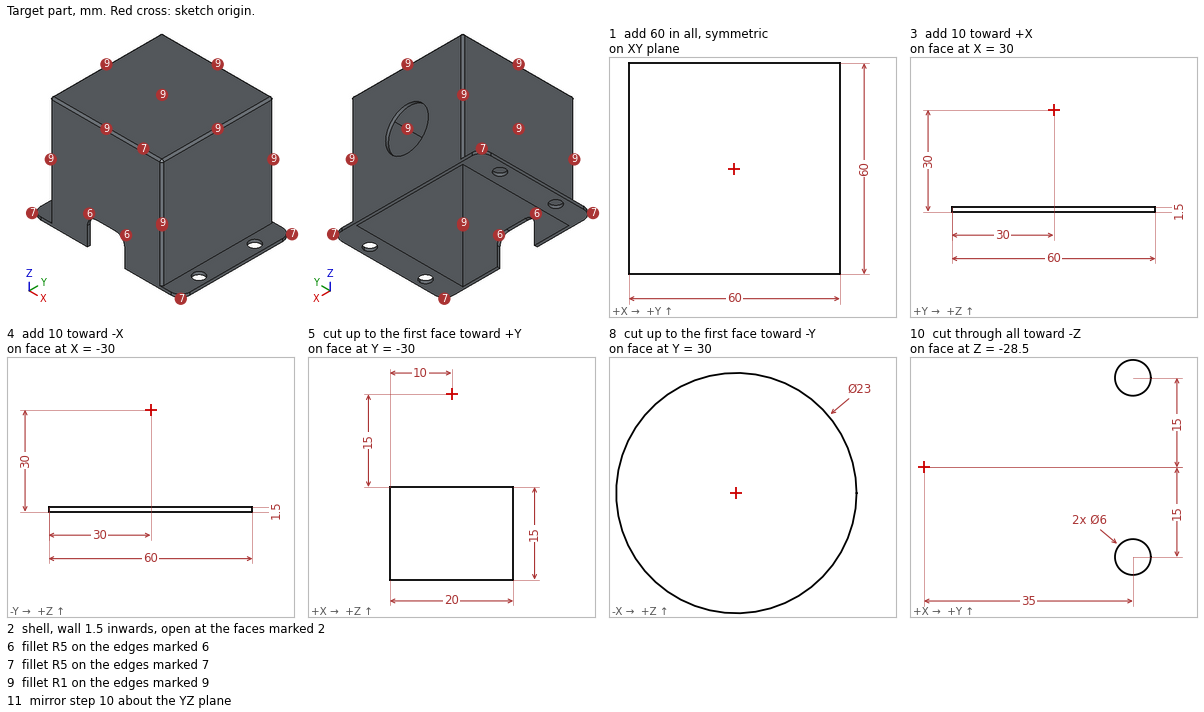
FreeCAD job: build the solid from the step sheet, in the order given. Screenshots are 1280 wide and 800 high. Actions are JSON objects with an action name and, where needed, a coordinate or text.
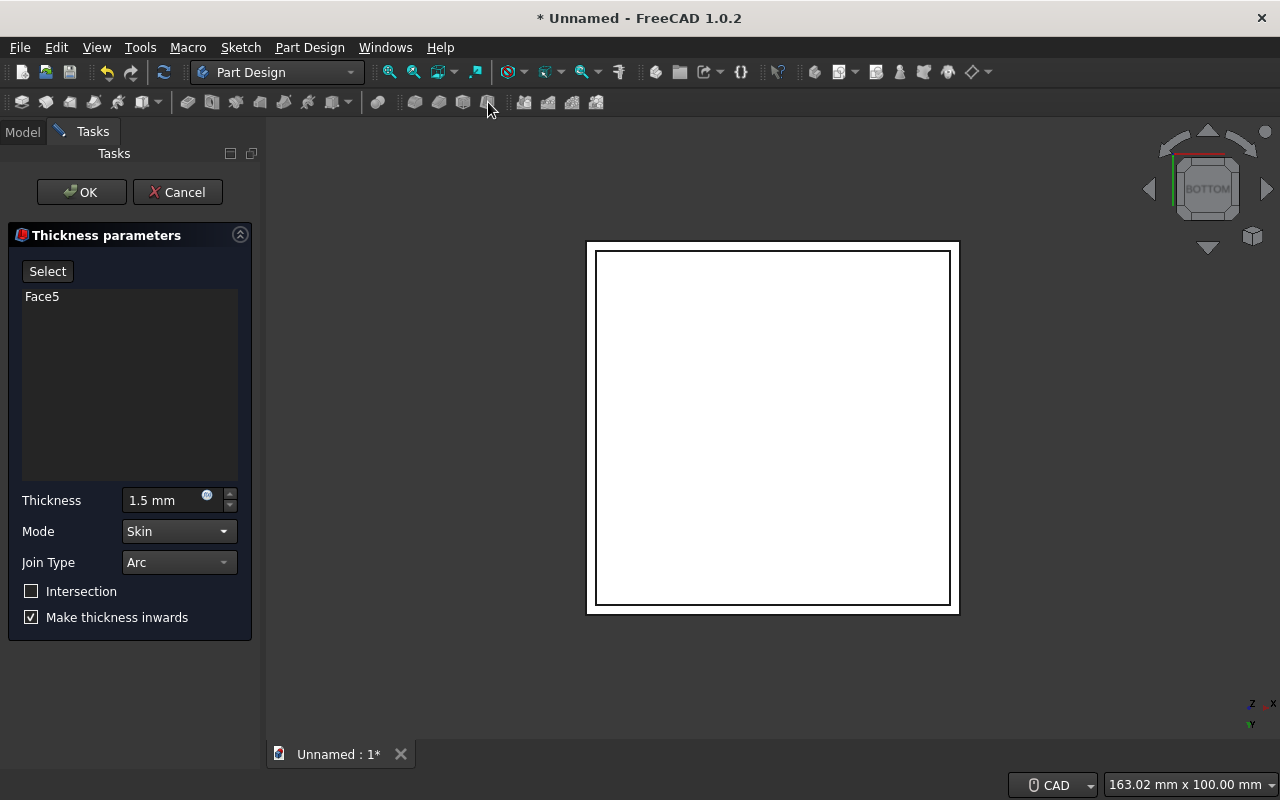
{"action": "left_click", "coordinate": [180, 562]}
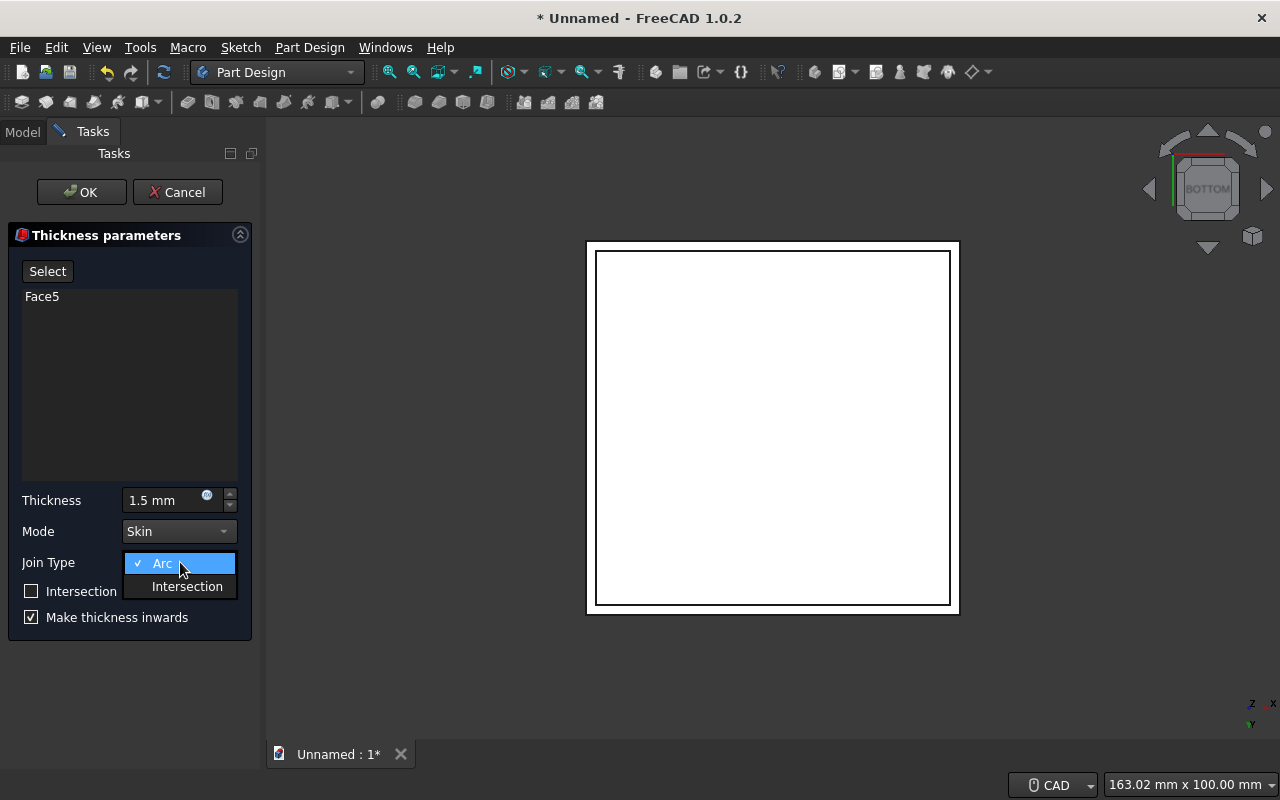
{"action": "left_click", "coordinate": [179, 586]}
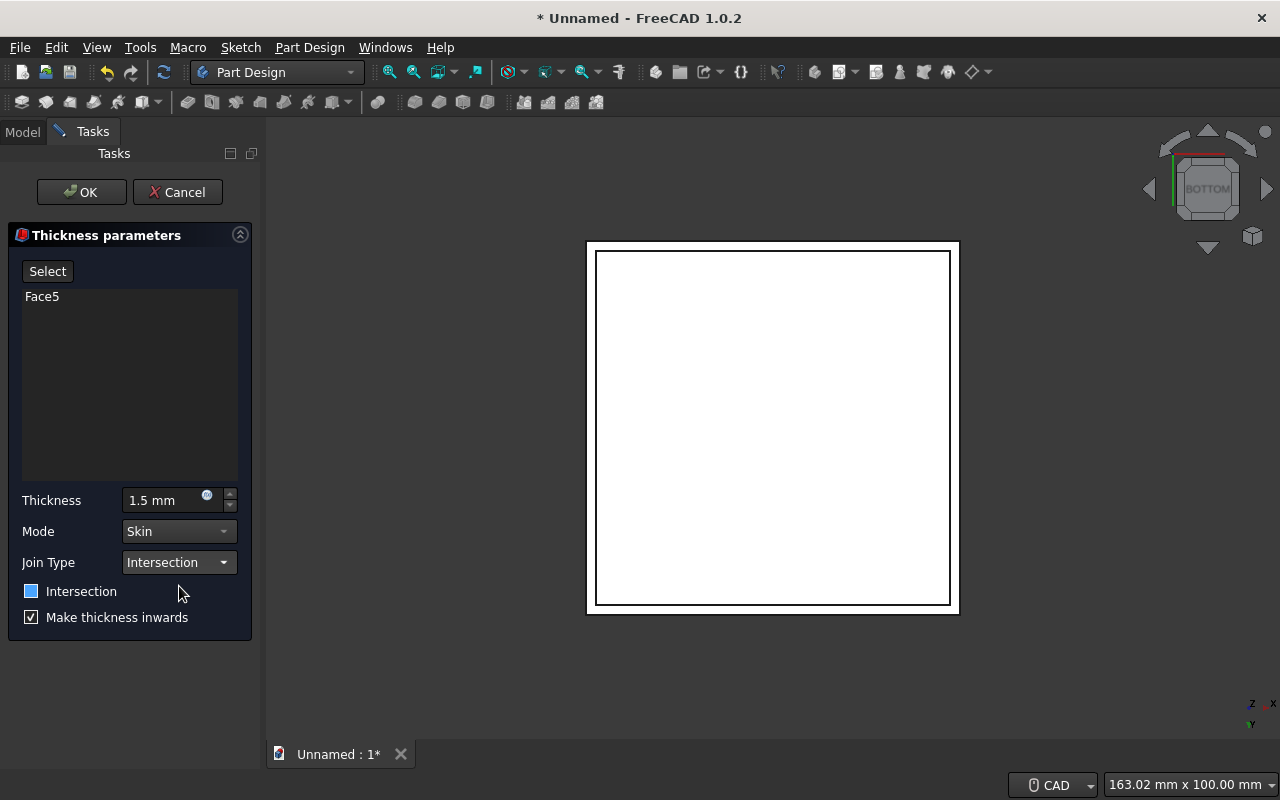
{"action": "left_click", "coordinate": [82, 192]}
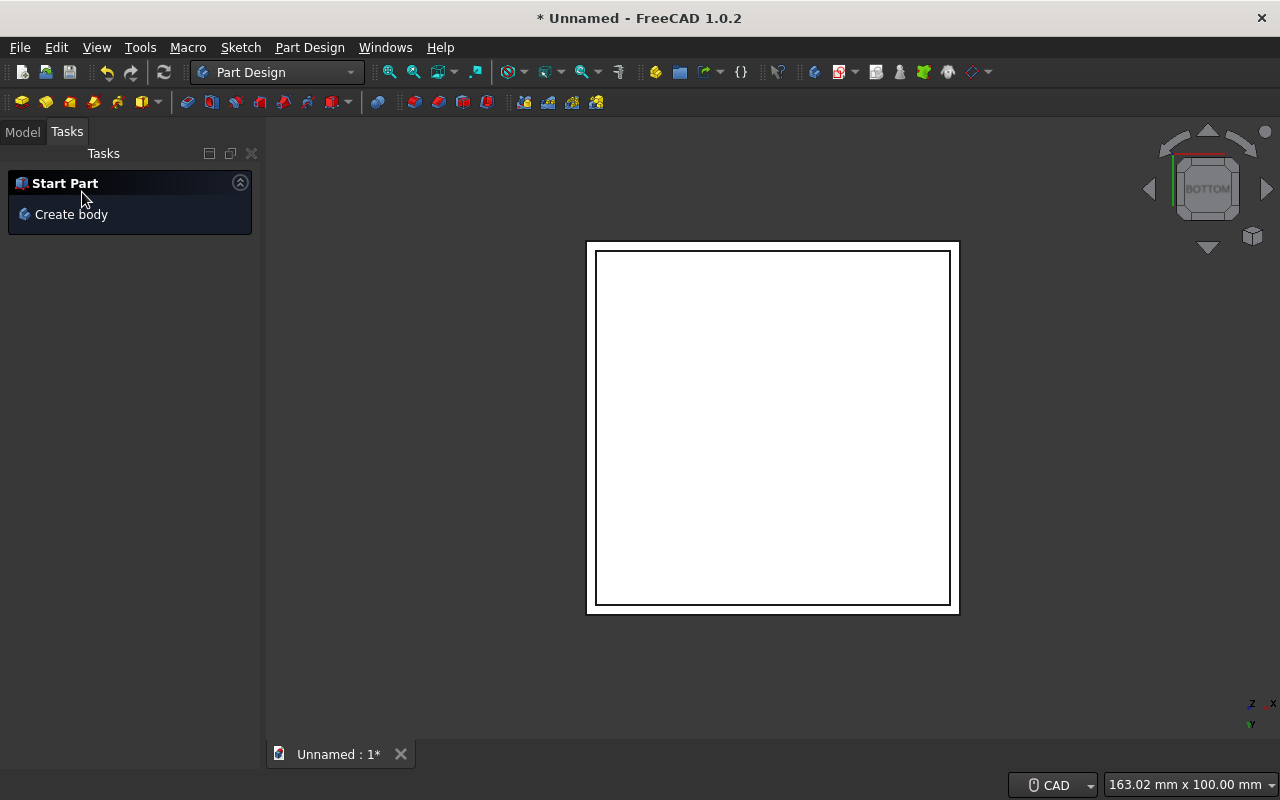
{"action": "key", "text": "0"}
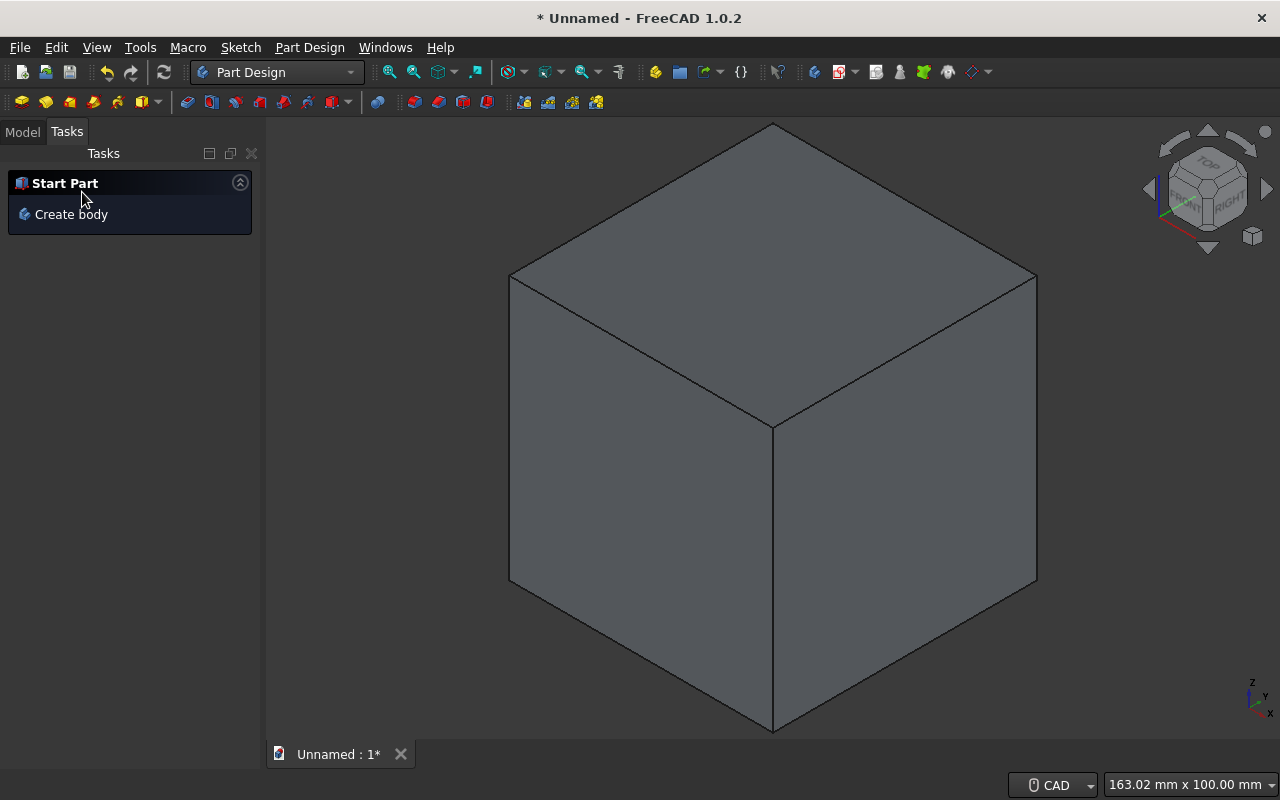
{"action": "left_click", "coordinate": [905, 503]}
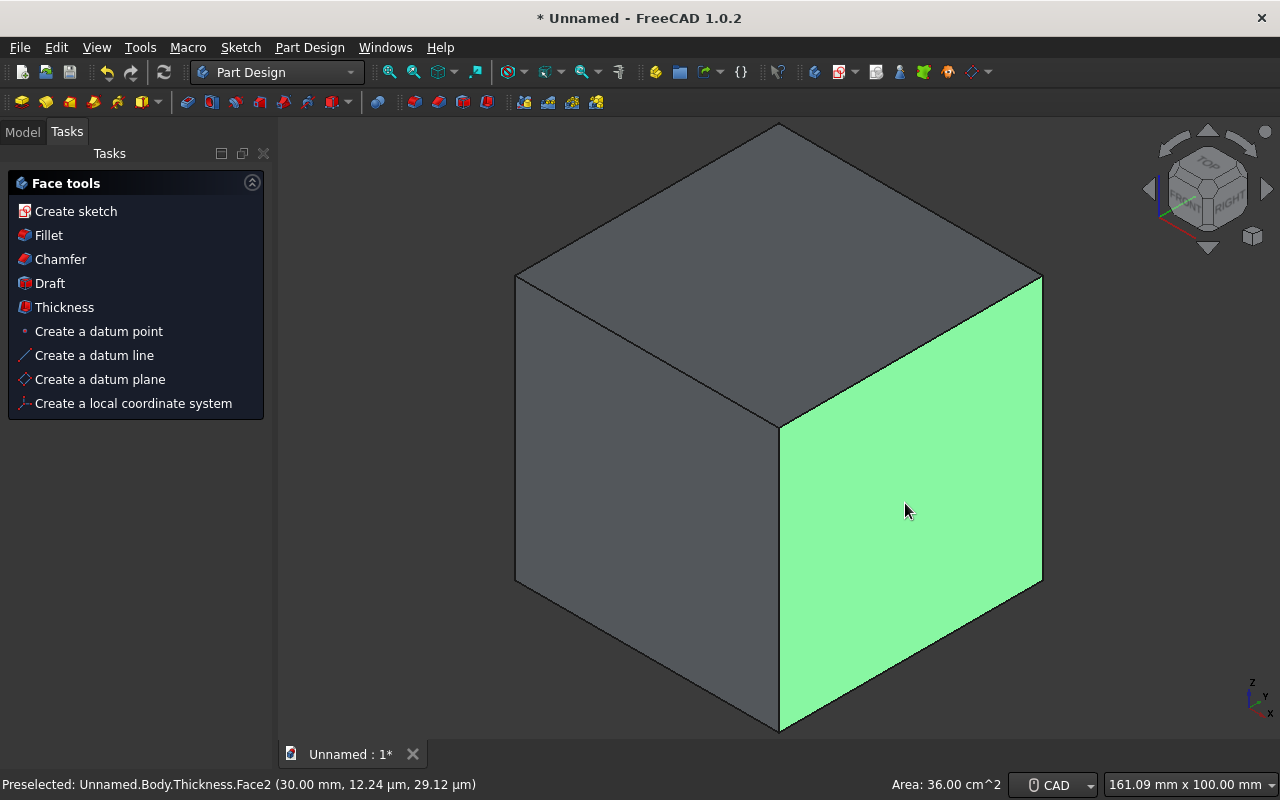
{"action": "left_click", "coordinate": [840, 72]}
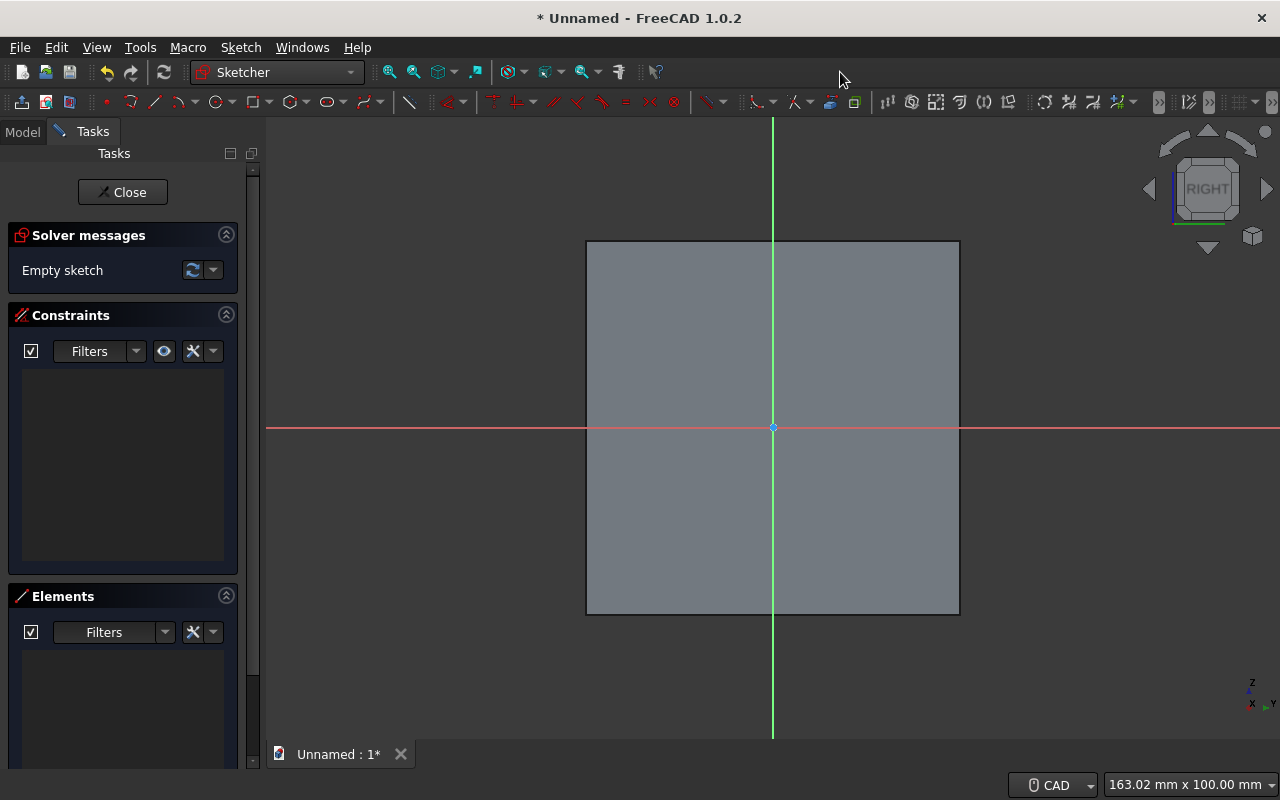
{"action": "scroll", "coordinate": [912, 711], "scroll_direction": "up", "scroll_amount": 2}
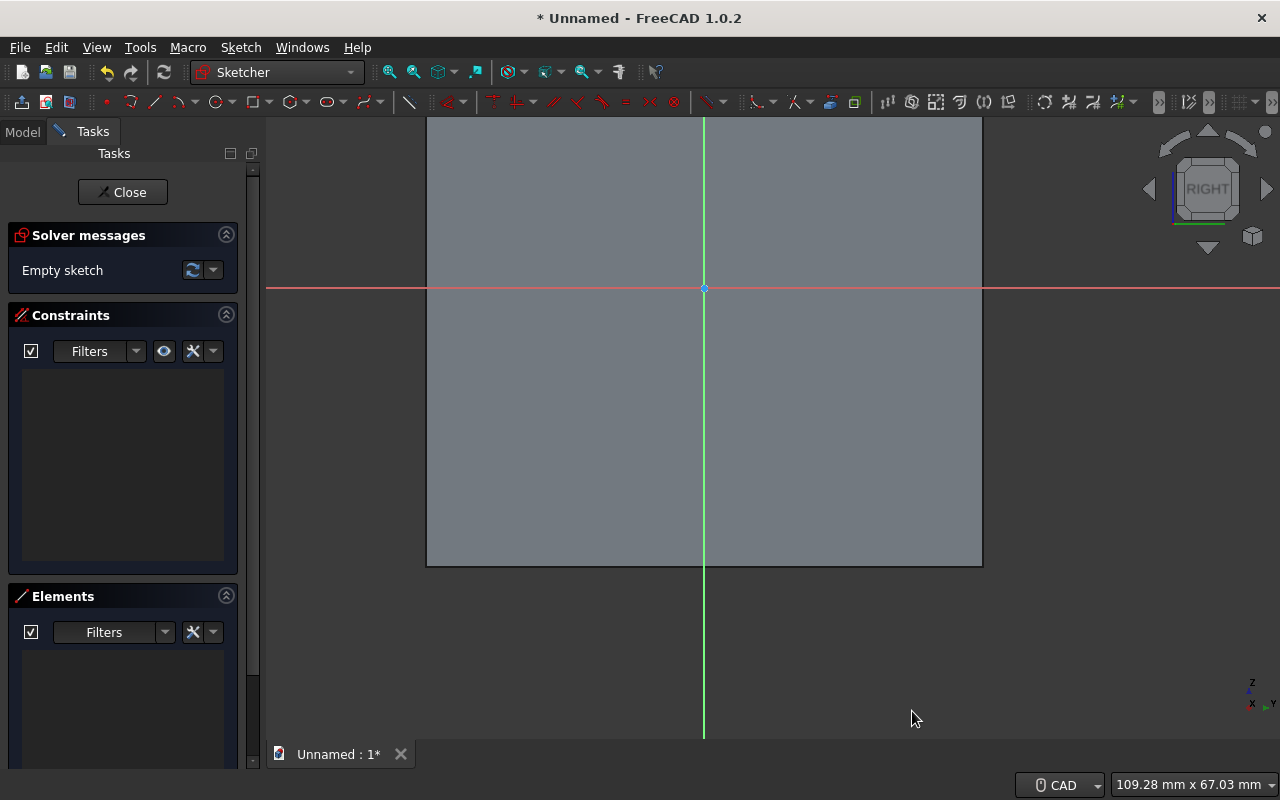
{"action": "key", "text": "g r"}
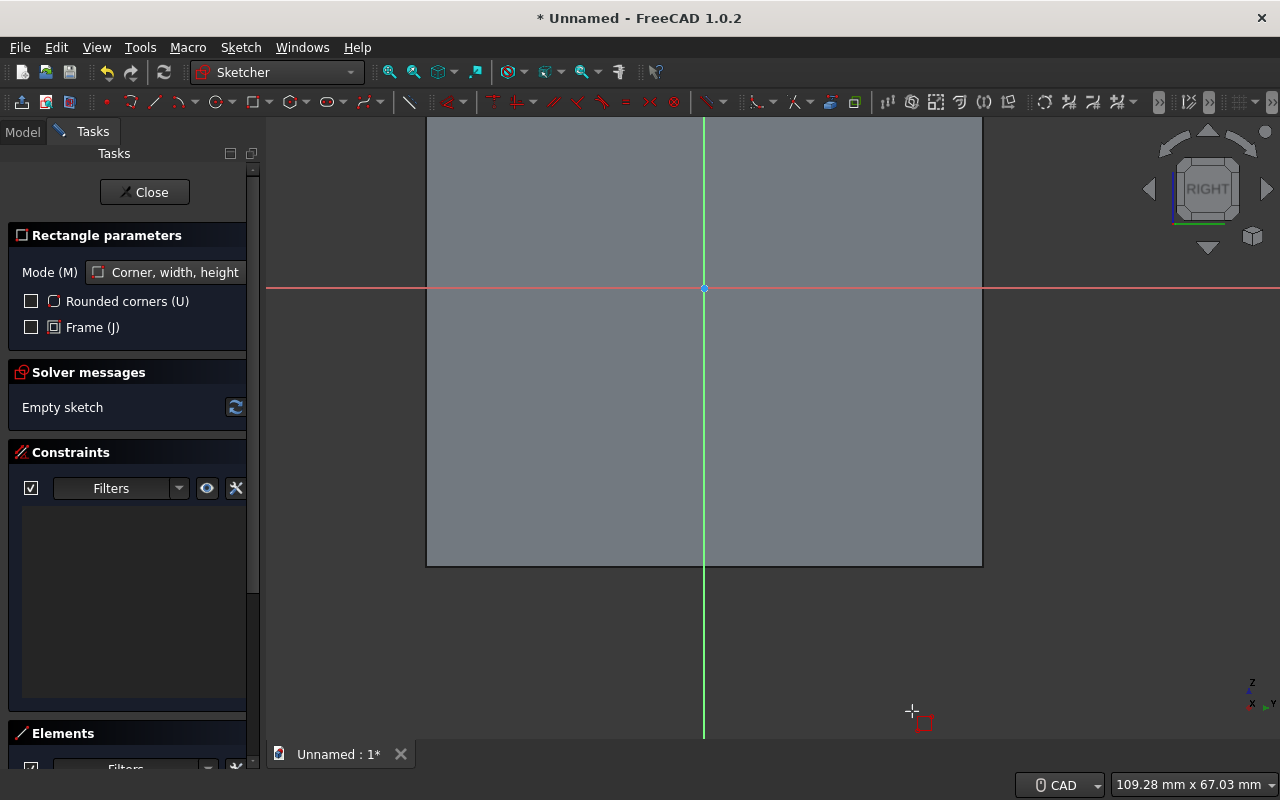
{"action": "left_click", "coordinate": [426, 553]}
{"action": "mouse_move", "coordinate": [983, 567]}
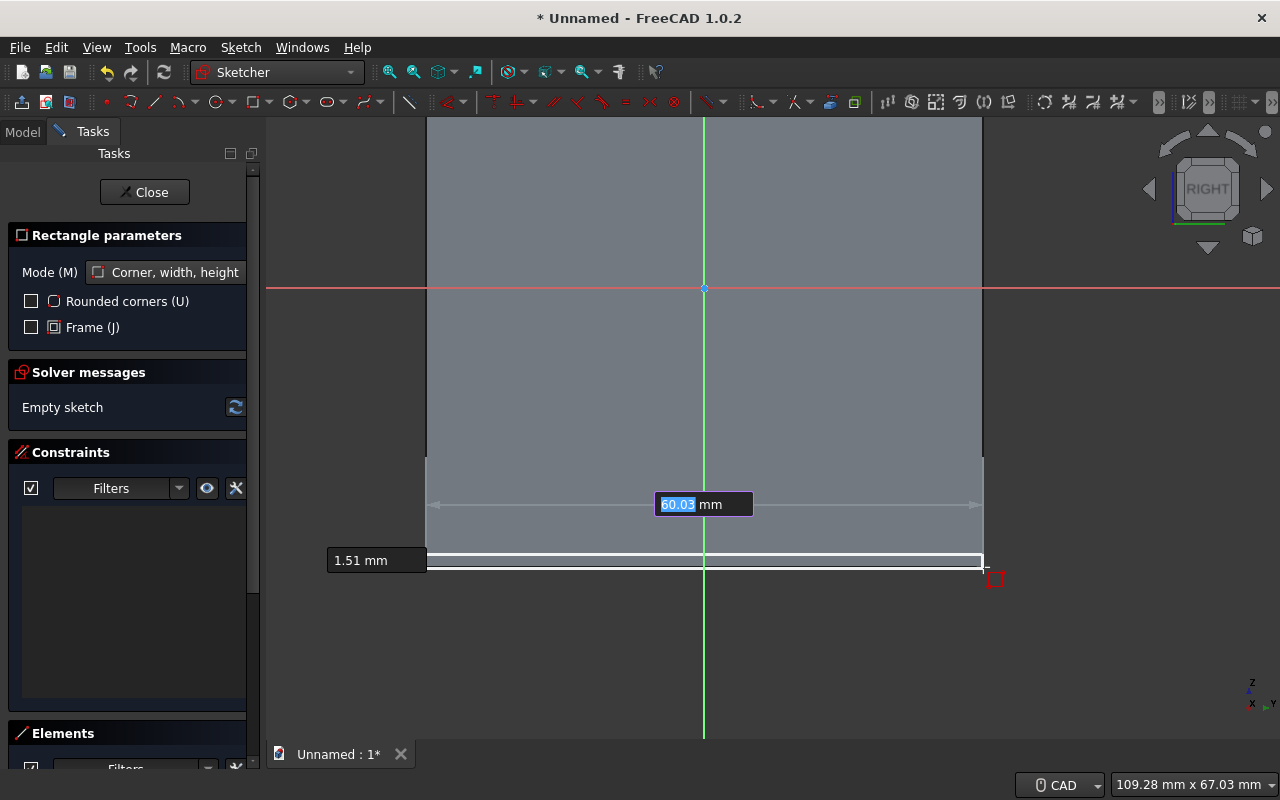
{"action": "type", "text": "60"}
{"action": "key", "text": "Tab"}
{"action": "type", "text": "1.5"}
{"action": "key", "text": "Return"}
{"action": "key", "text": "Escape"}